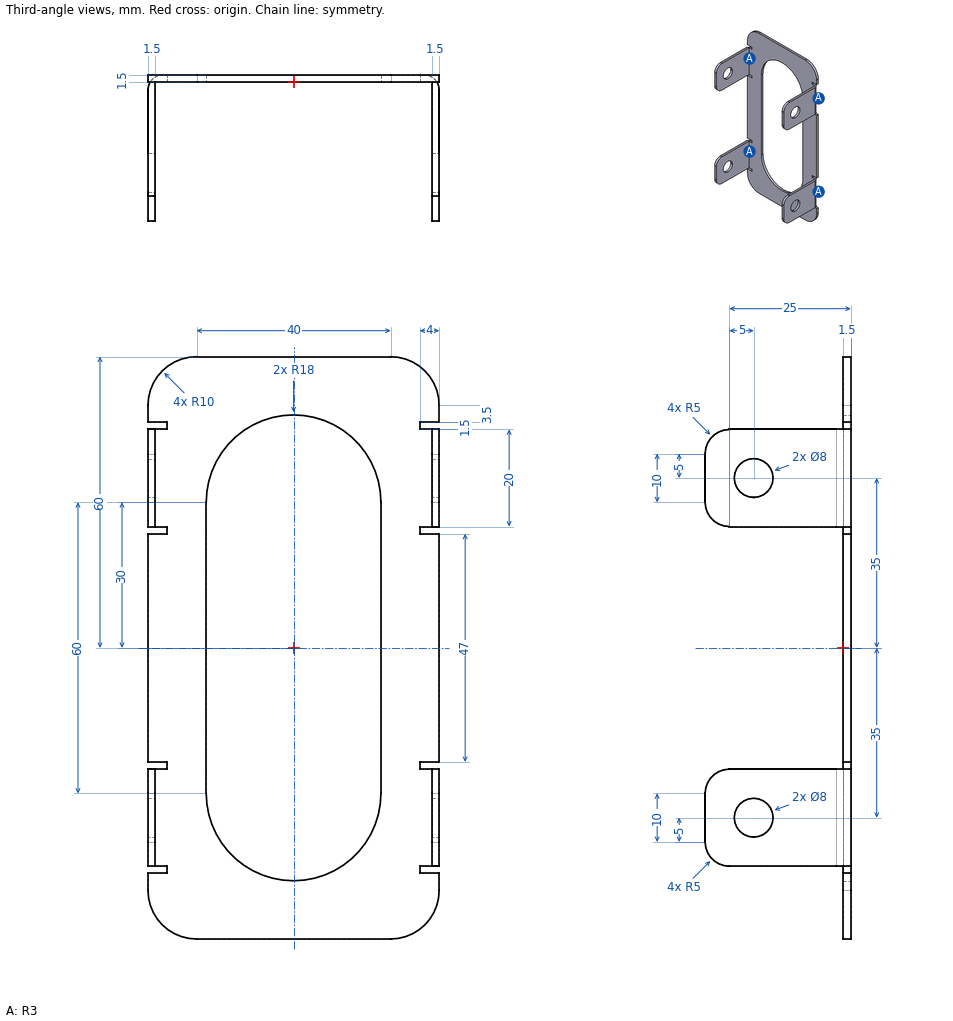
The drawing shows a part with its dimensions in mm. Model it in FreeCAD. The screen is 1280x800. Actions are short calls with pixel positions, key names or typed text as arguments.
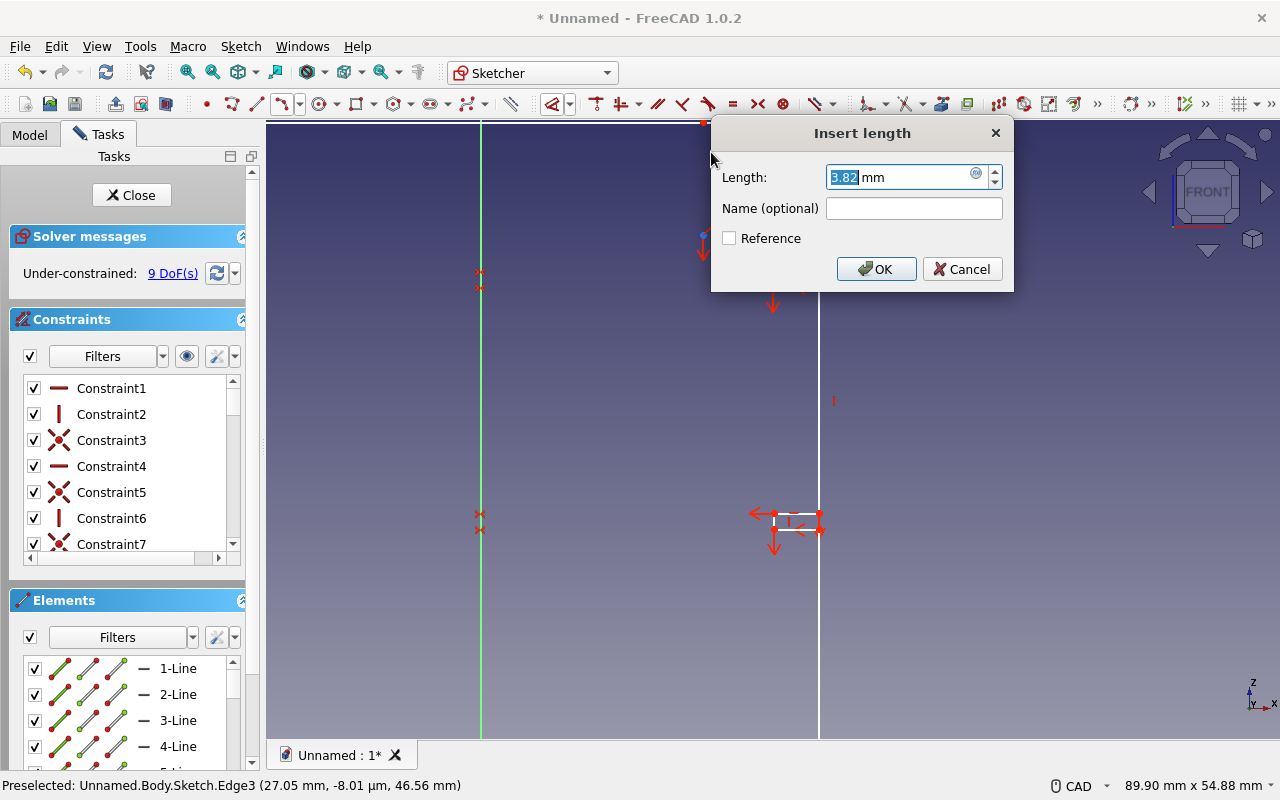
text(4)
key(Return)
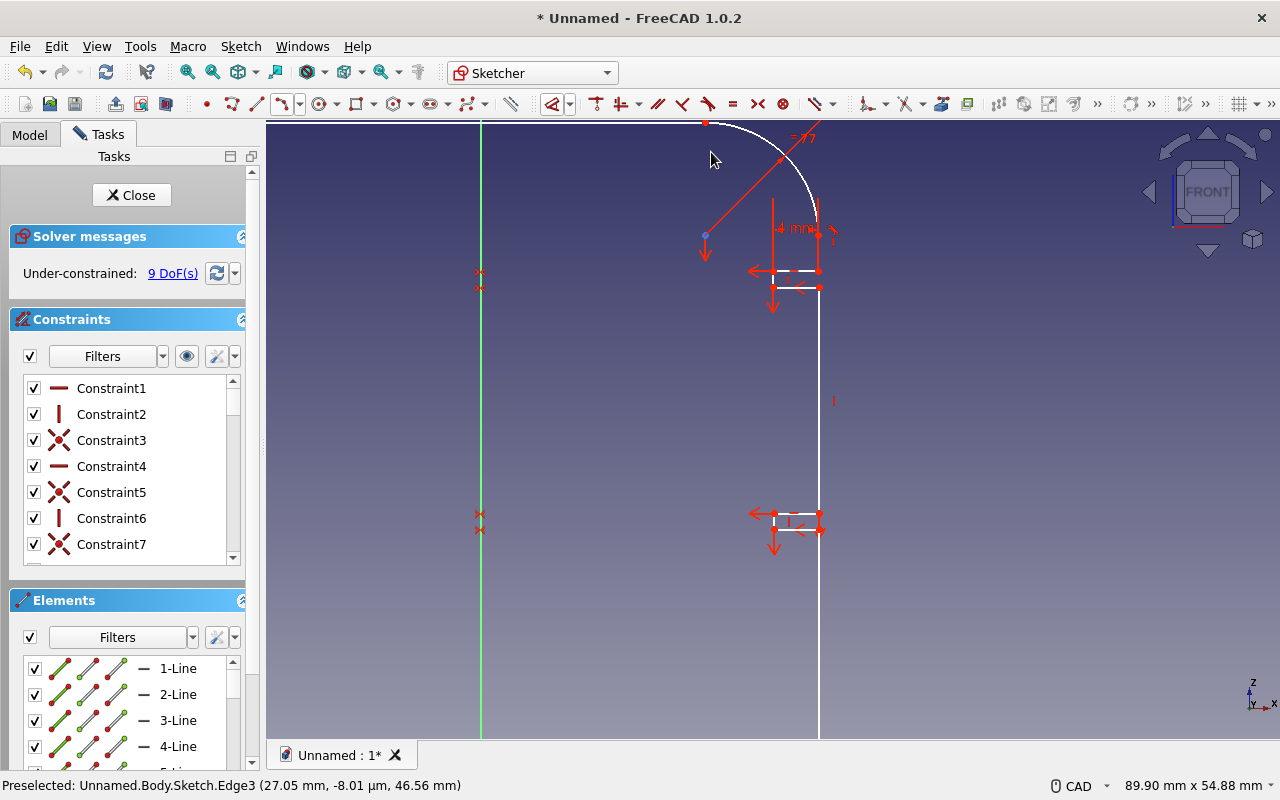
click(787, 288)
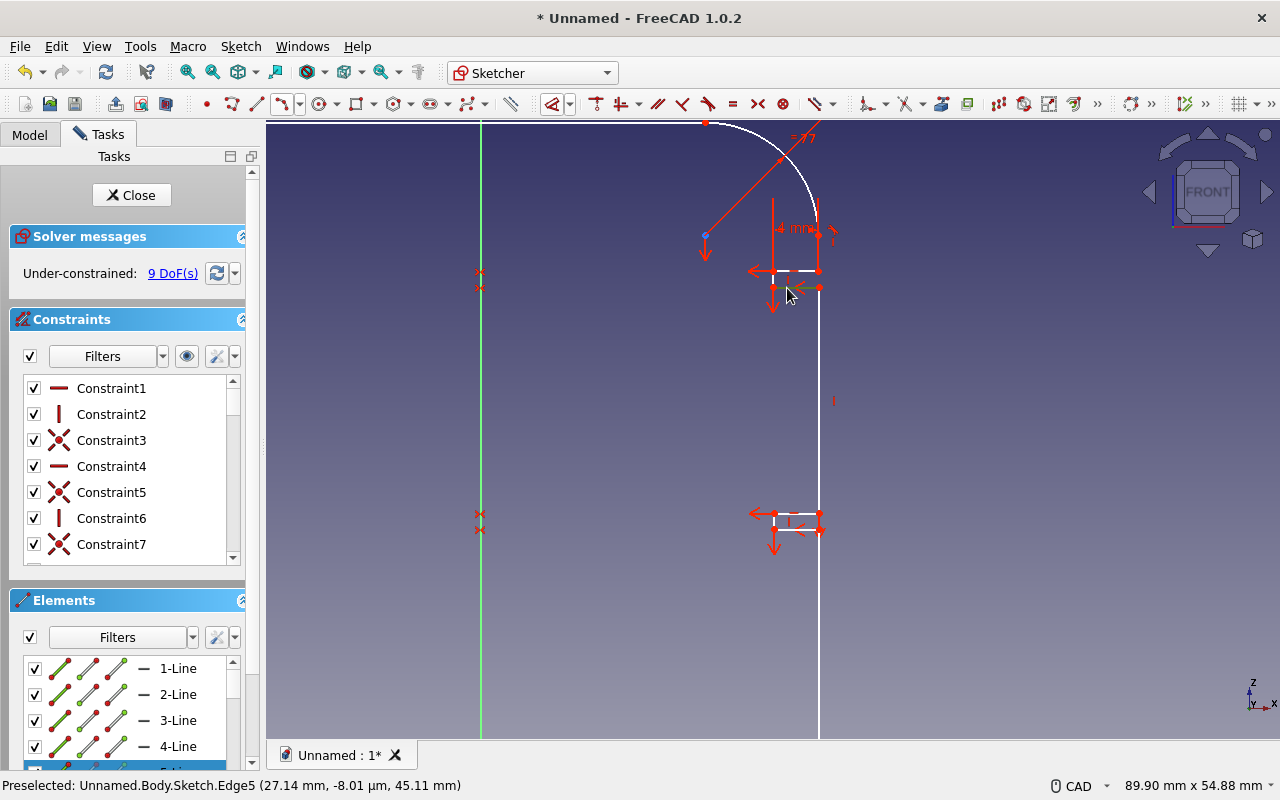
click(570, 104)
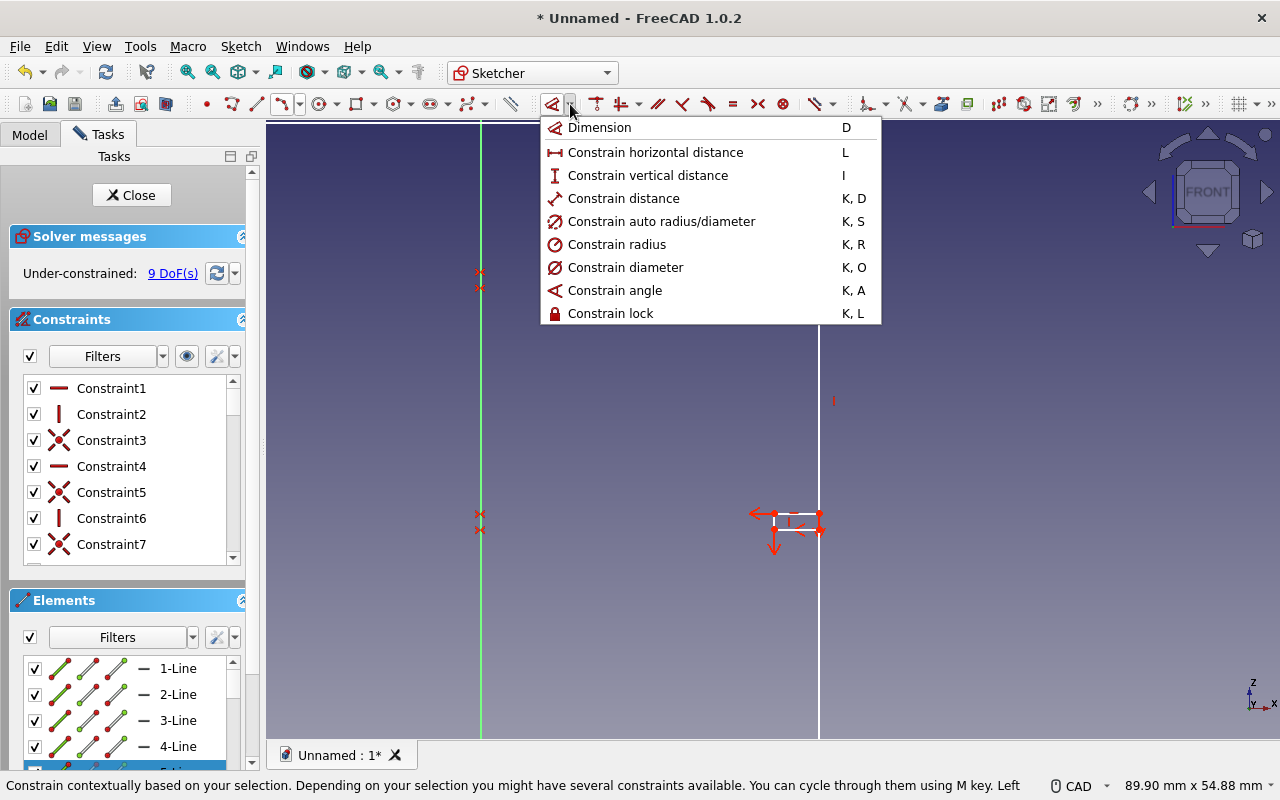
click(711, 152)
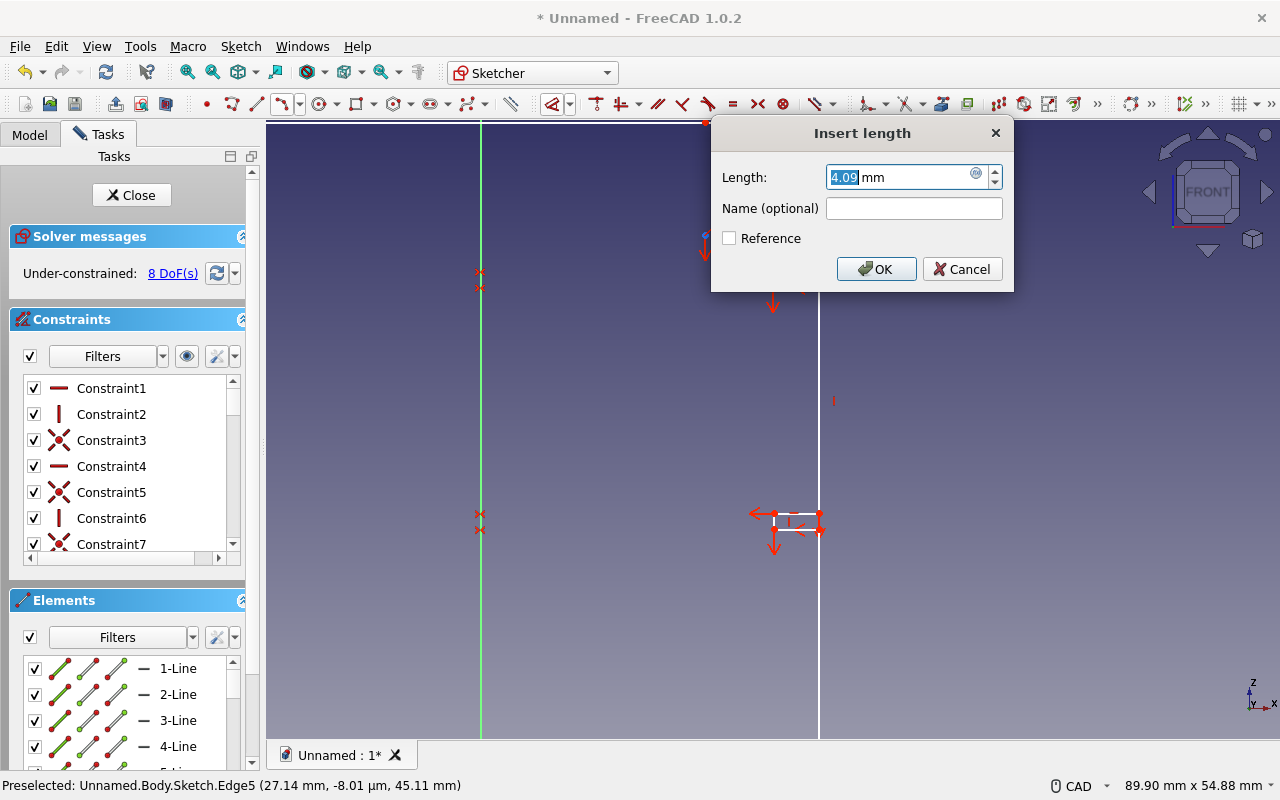
text(4)
key(Return)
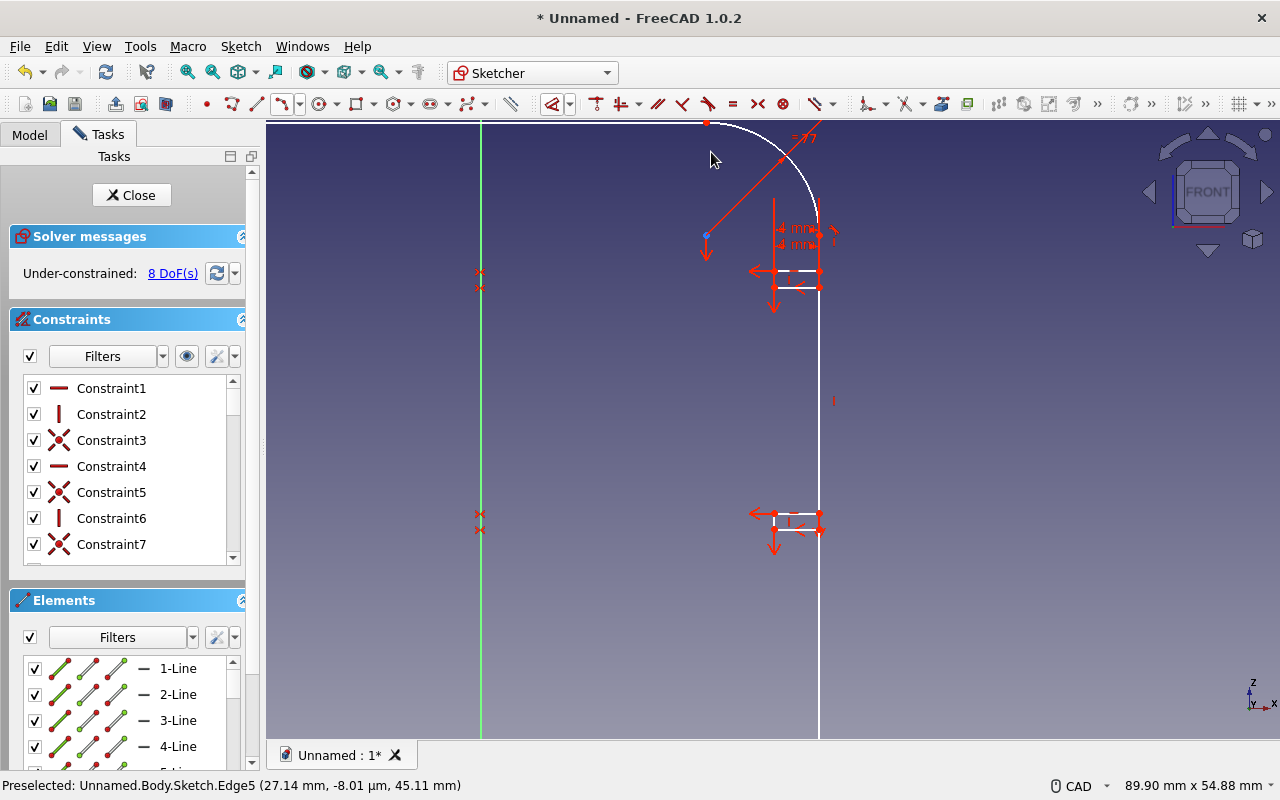
click(806, 514)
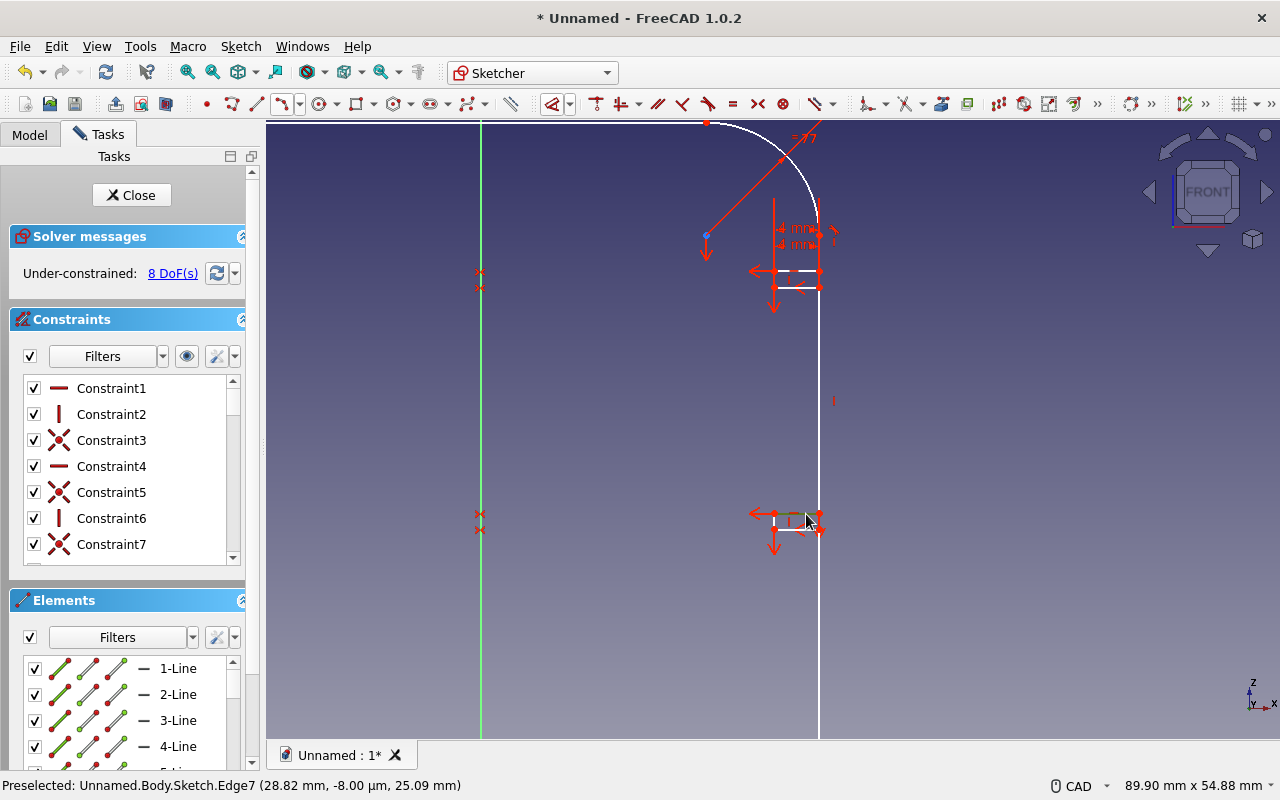
key(l)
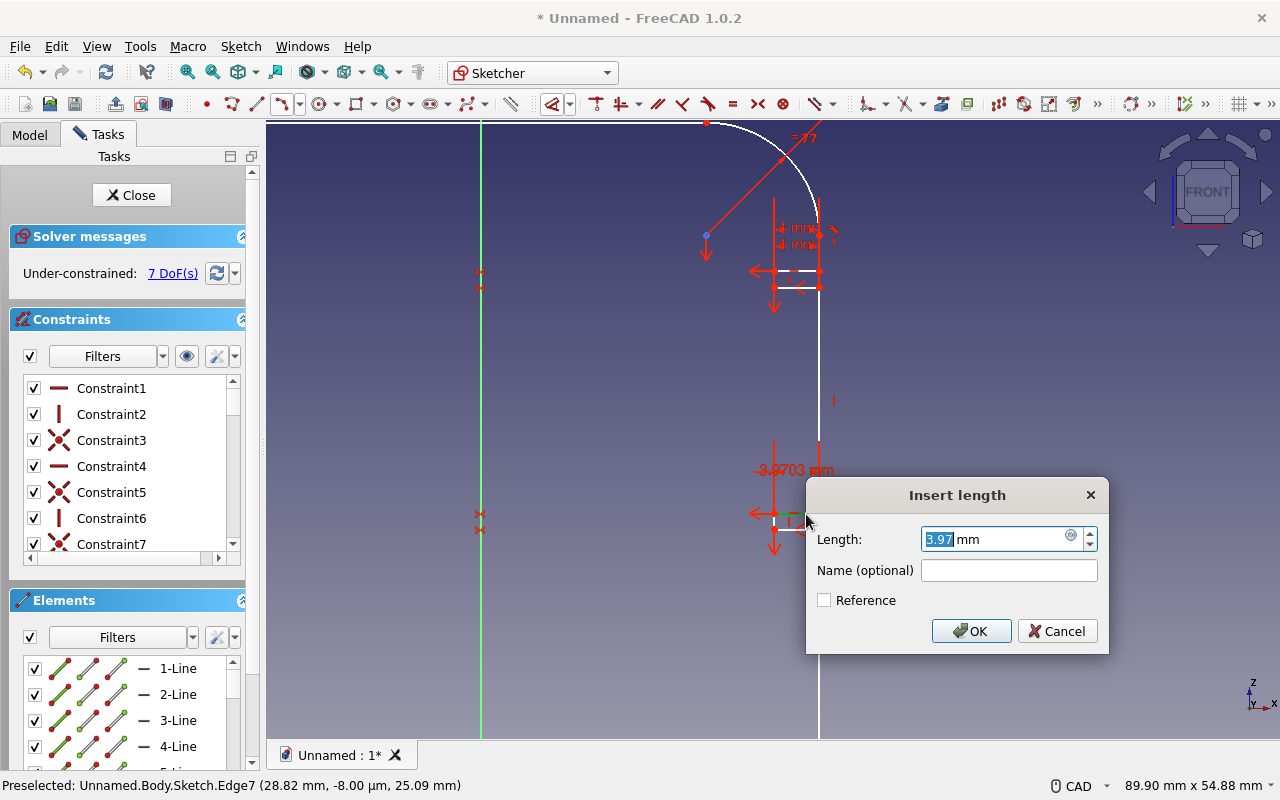
text(4)
key(Return)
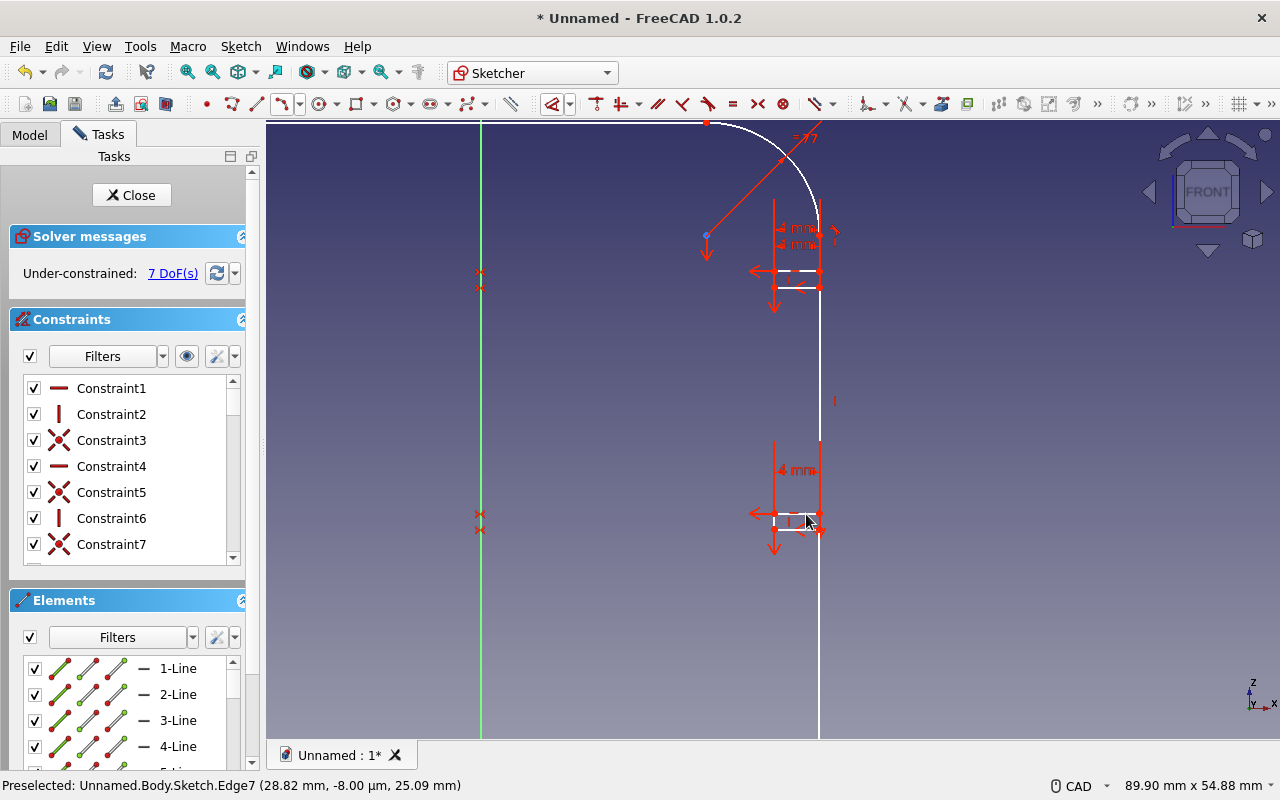
click(788, 530)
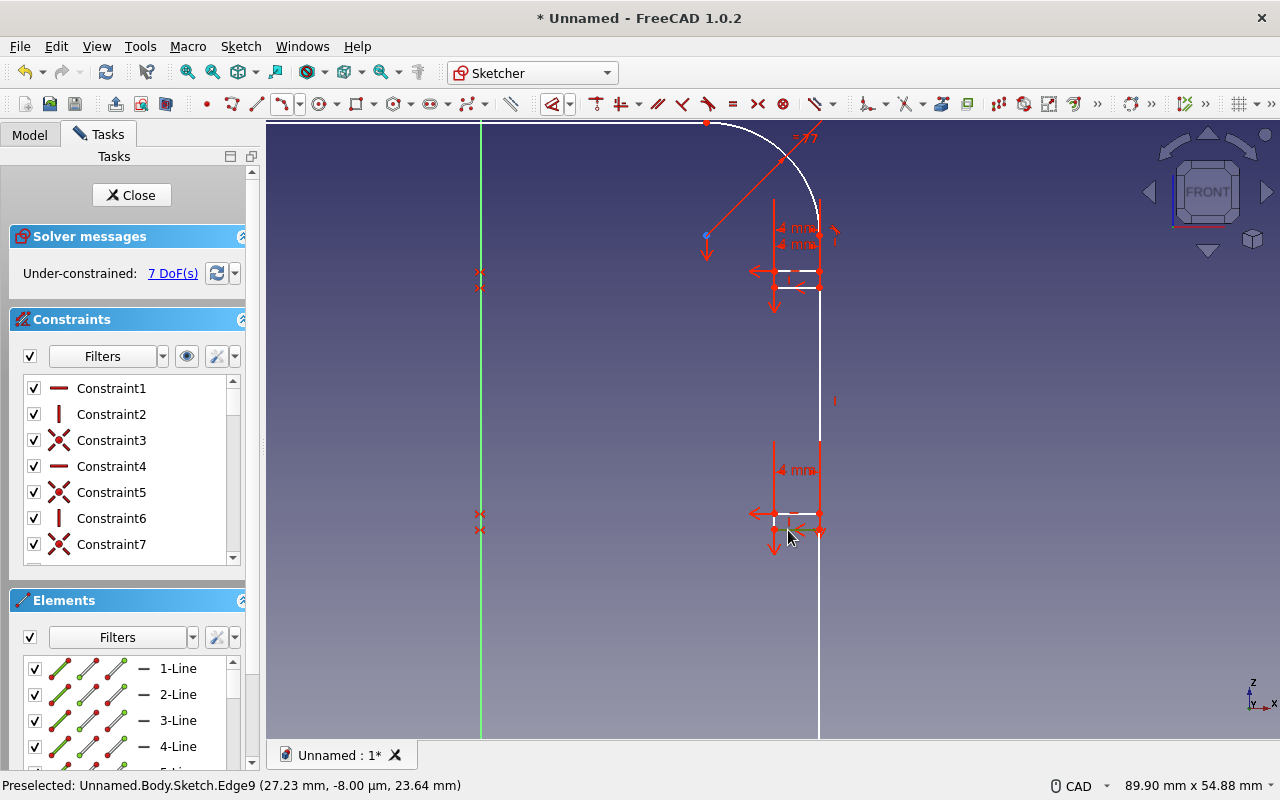
click(570, 104)